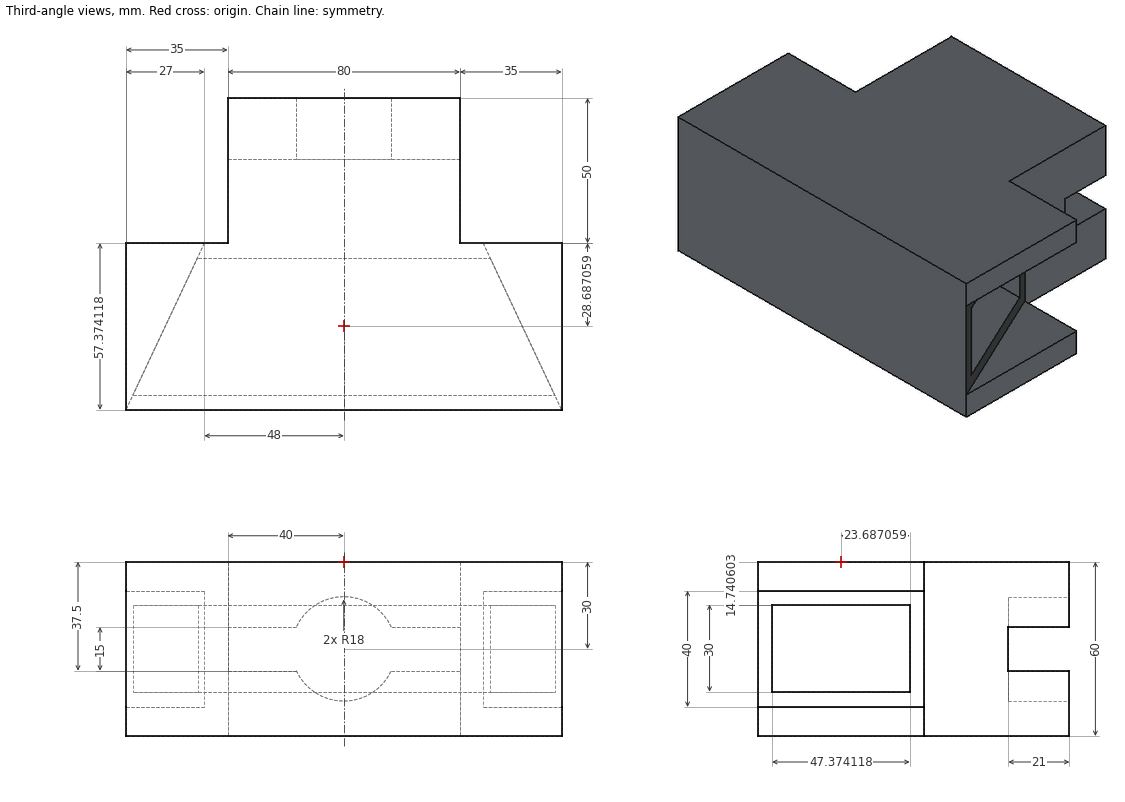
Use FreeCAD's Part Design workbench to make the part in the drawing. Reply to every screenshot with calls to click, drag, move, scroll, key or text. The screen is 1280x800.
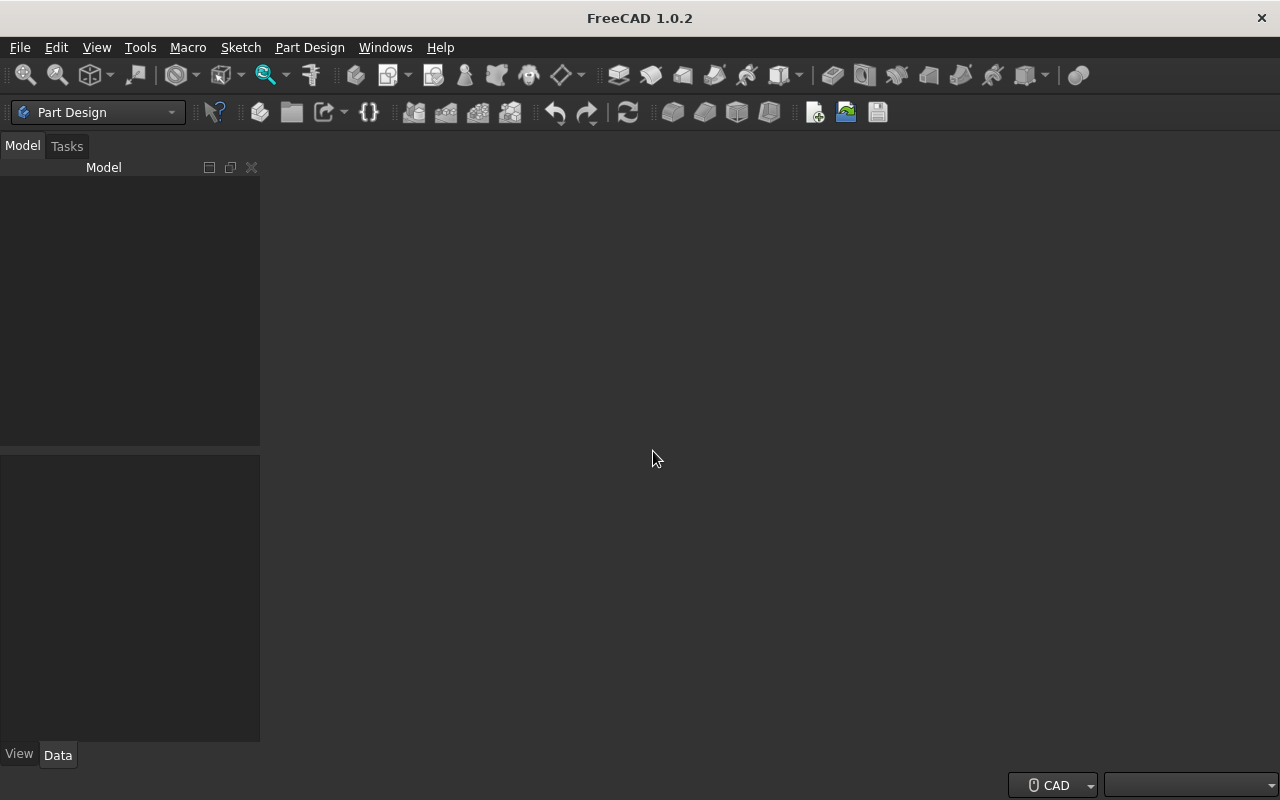
key(ctrl+n)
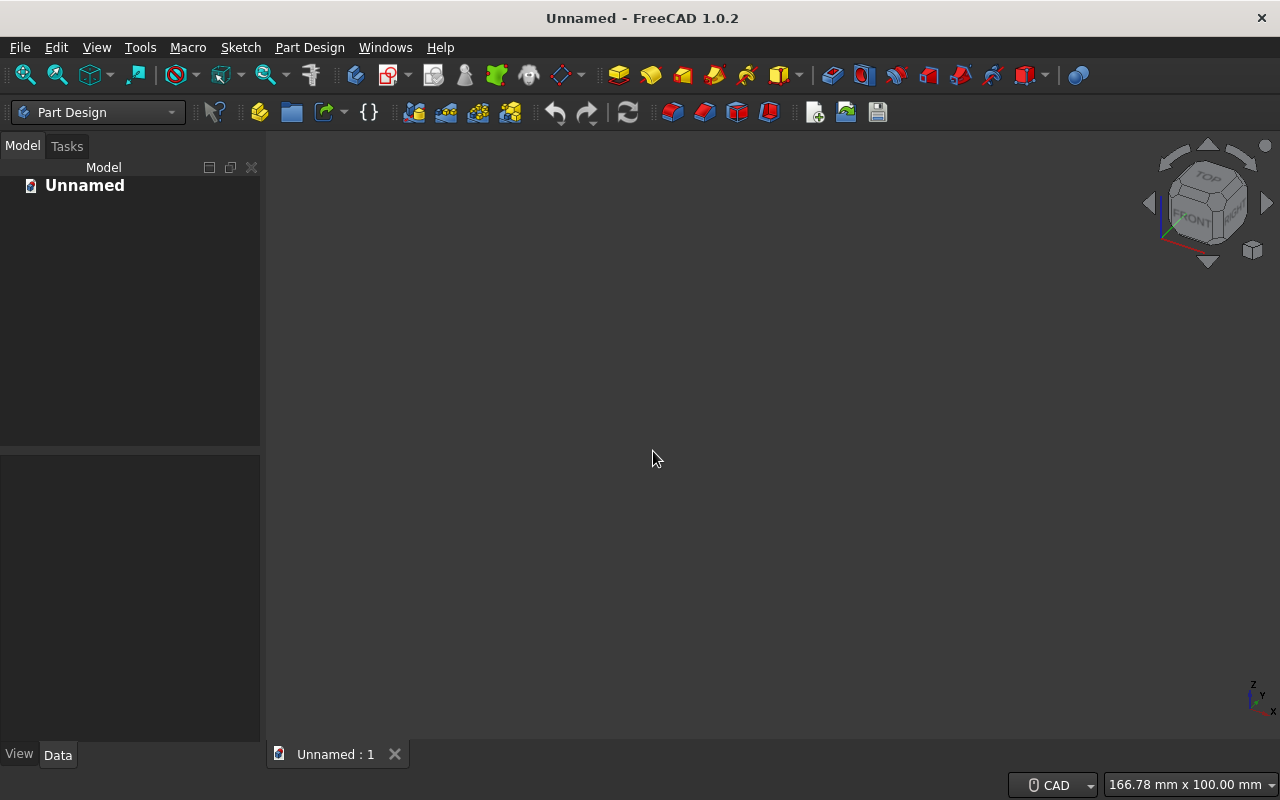
click(388, 76)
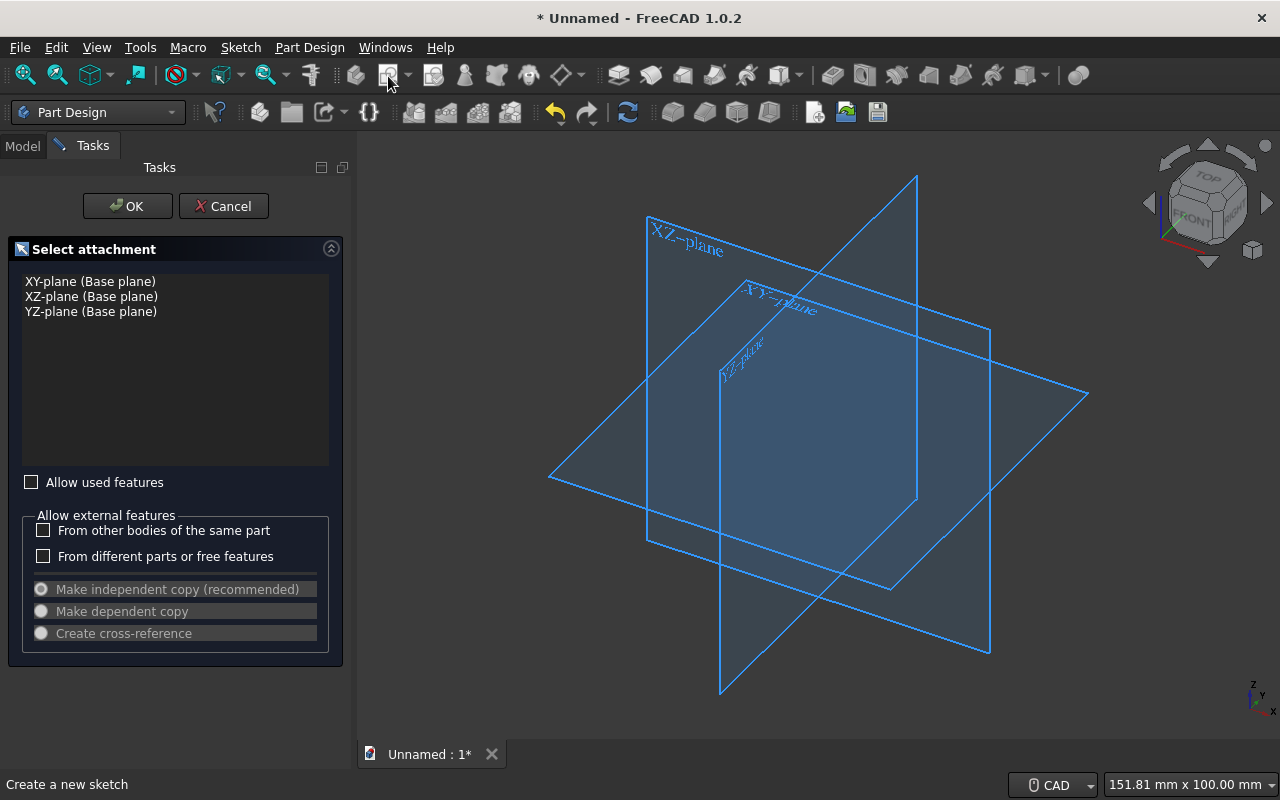
click(82, 282)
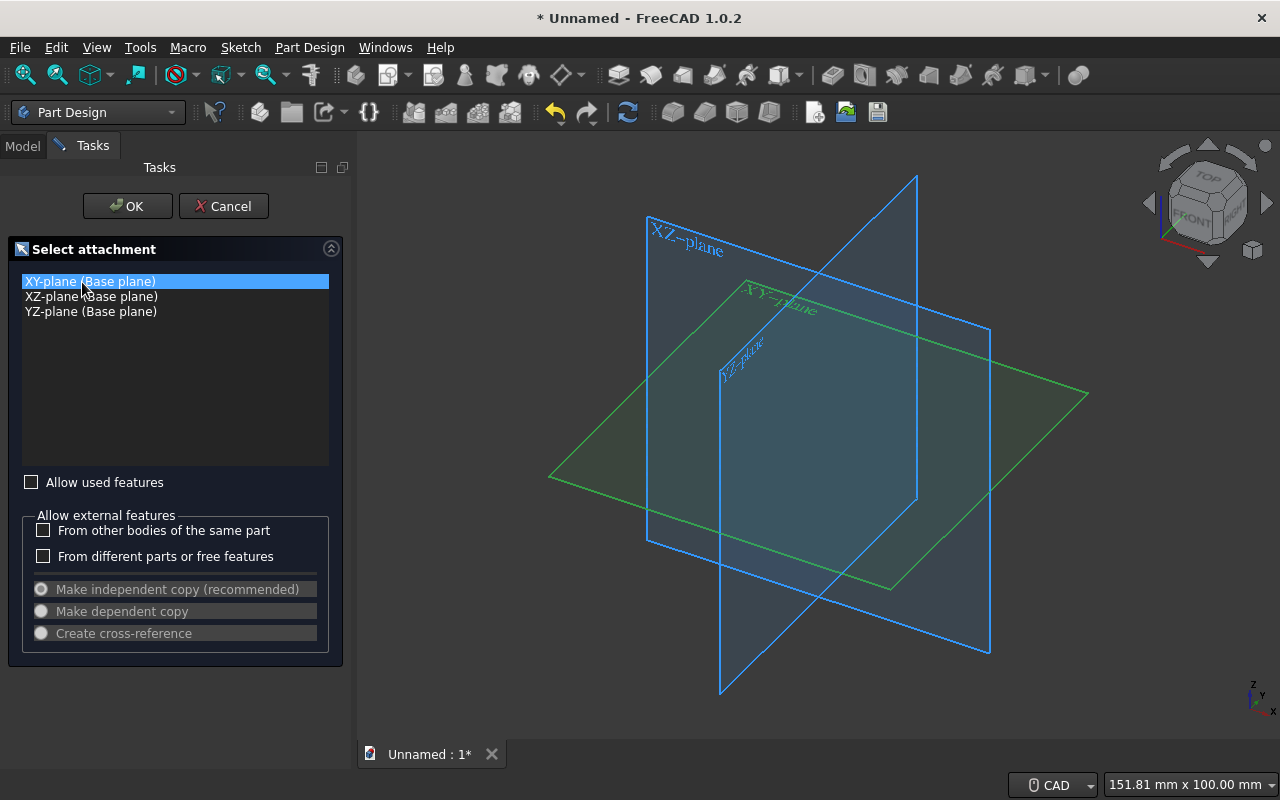
click(128, 206)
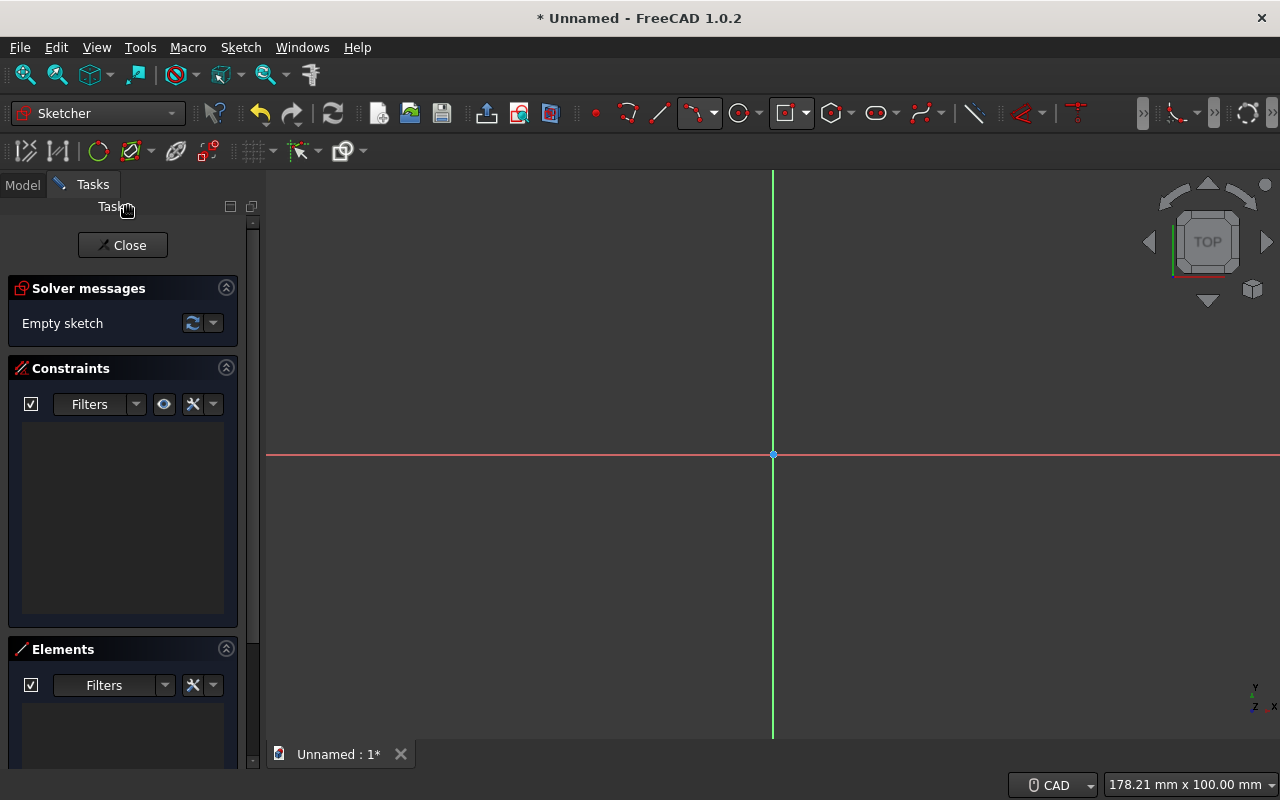
scroll(621, 628, down, 3)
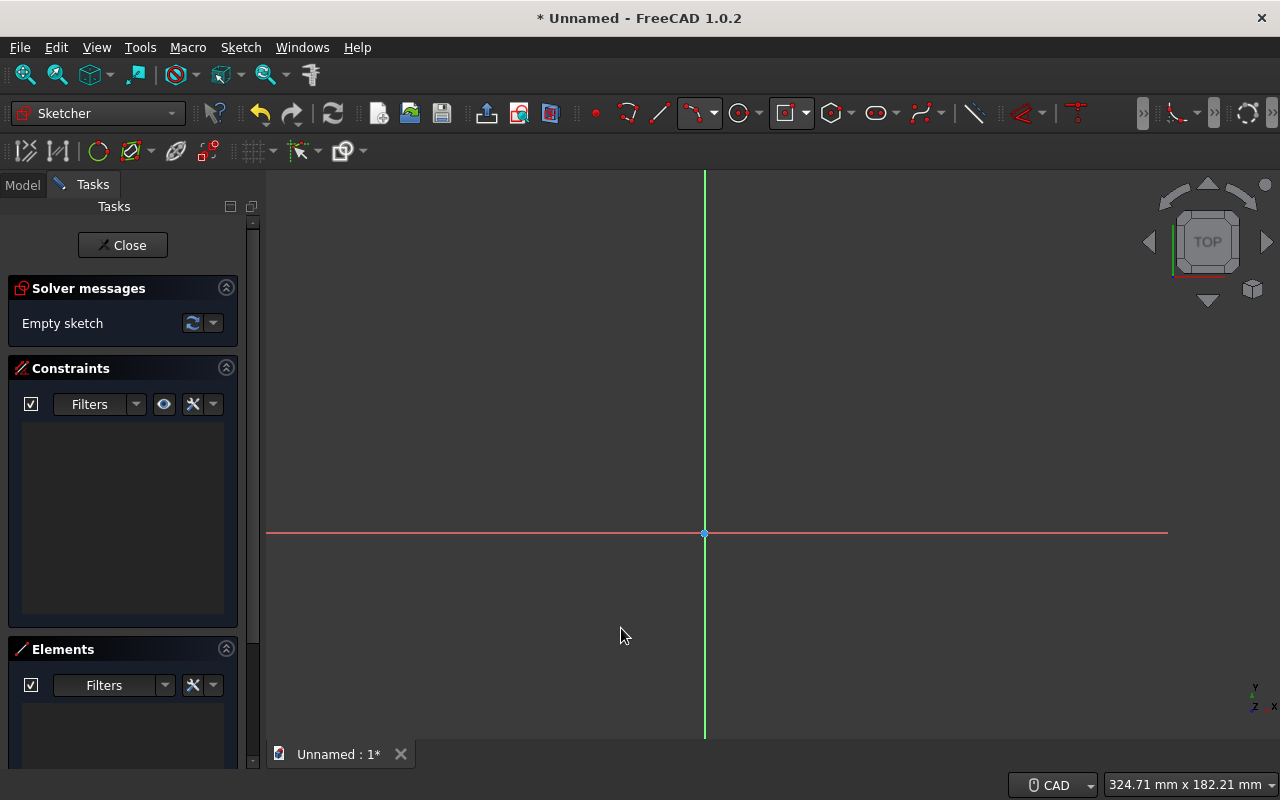
key(g)
key(m)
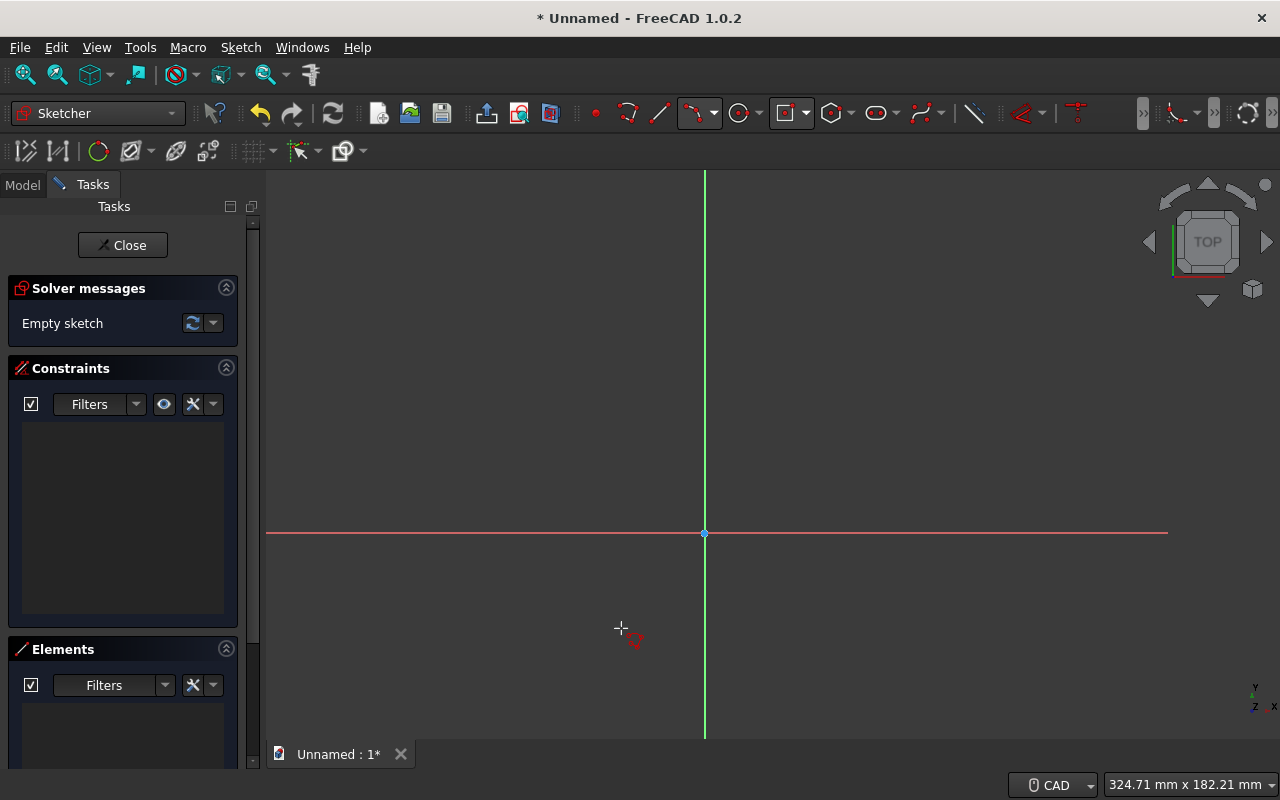
click(829, 444)
click(829, 287)
click(580, 287)
click(580, 444)
click(470, 444)
click(470, 623)
click(939, 623)
click(939, 444)
click(829, 445)
key(Escape)
key(Escape)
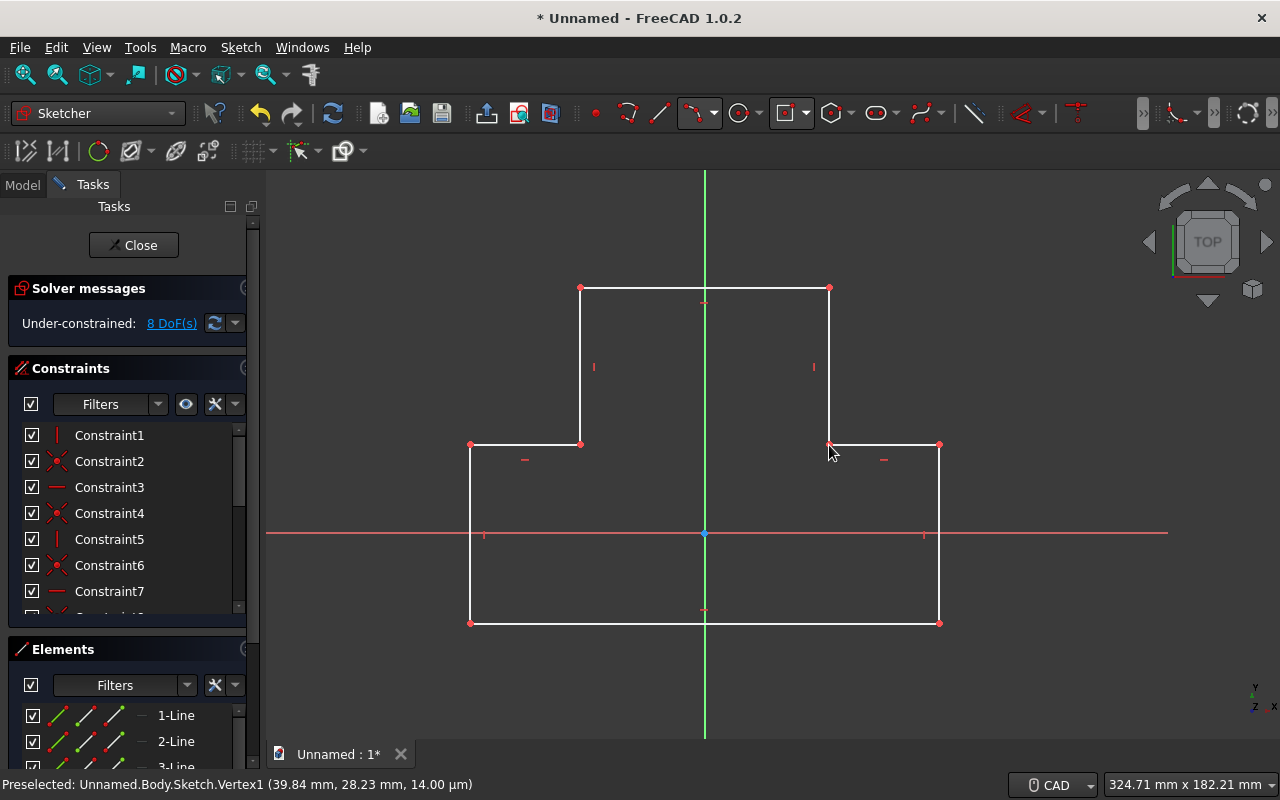
click(829, 445)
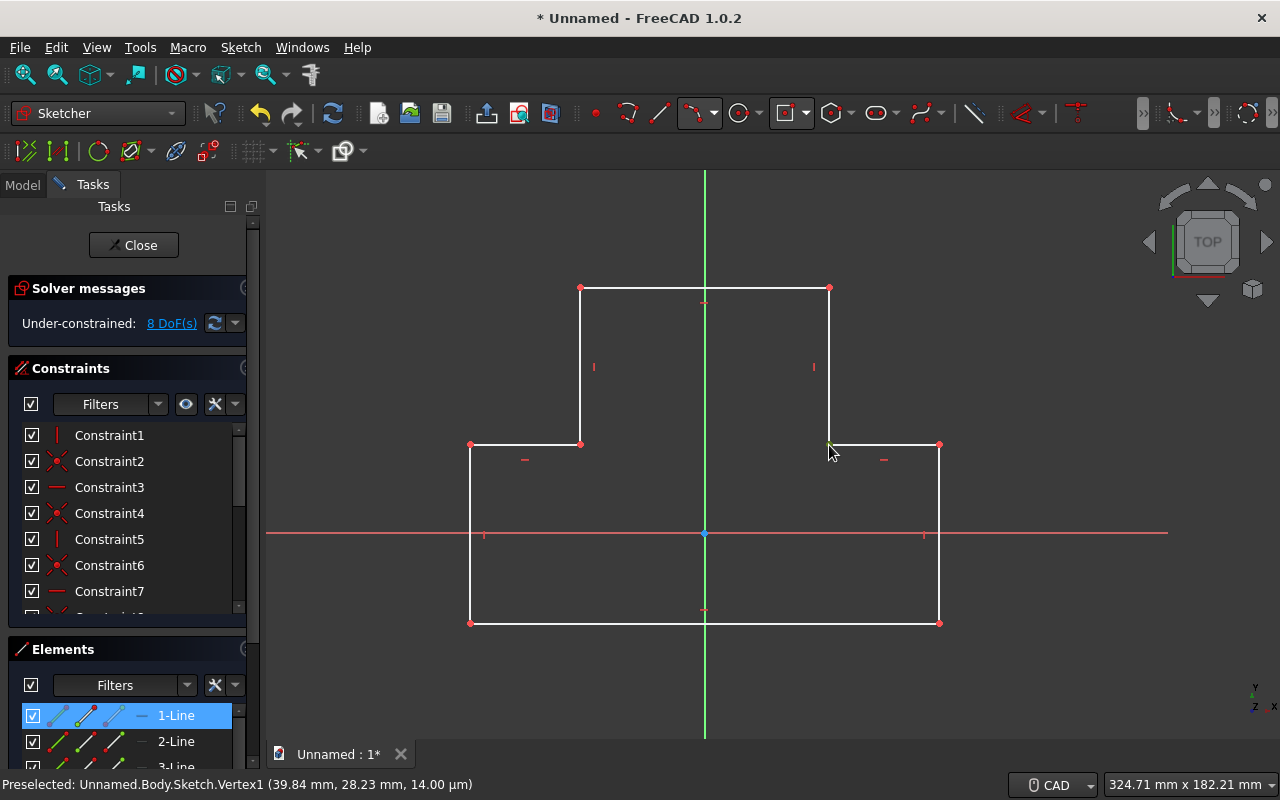
click(580, 445)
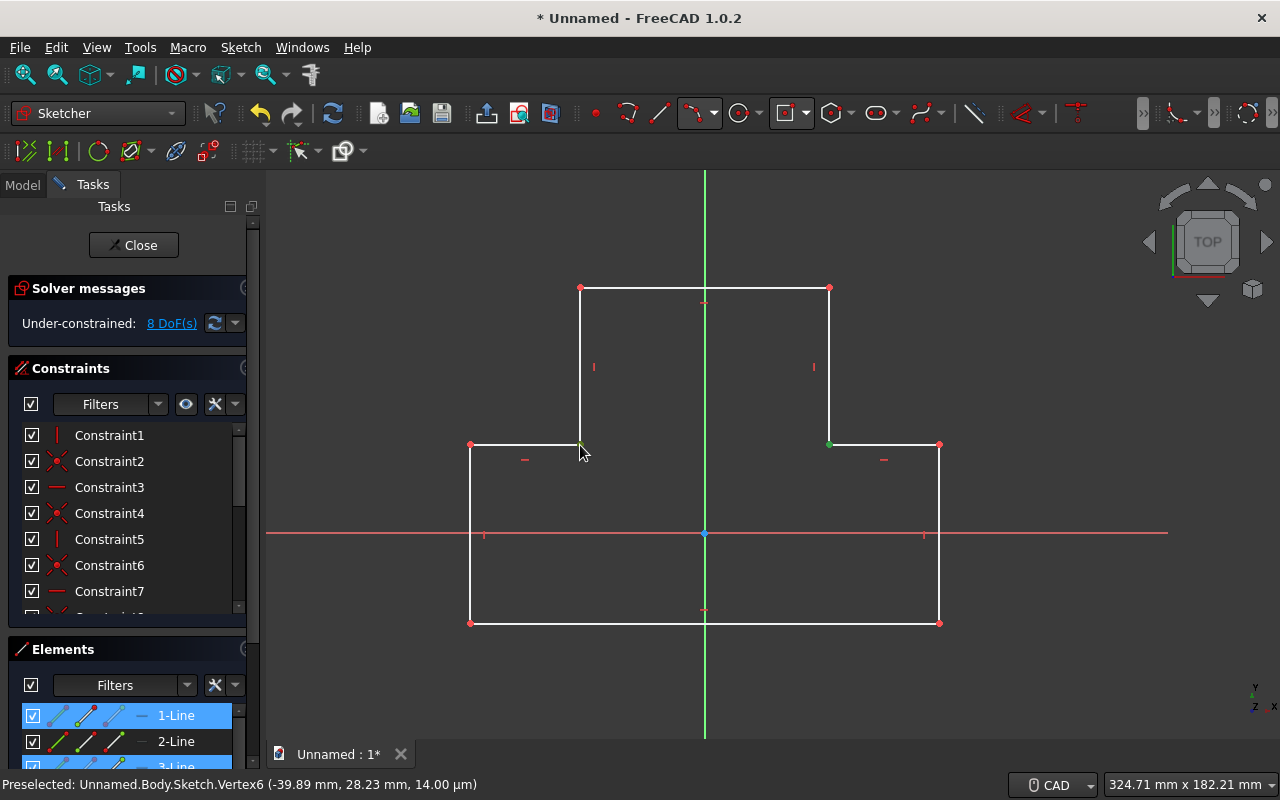
click(705, 674)